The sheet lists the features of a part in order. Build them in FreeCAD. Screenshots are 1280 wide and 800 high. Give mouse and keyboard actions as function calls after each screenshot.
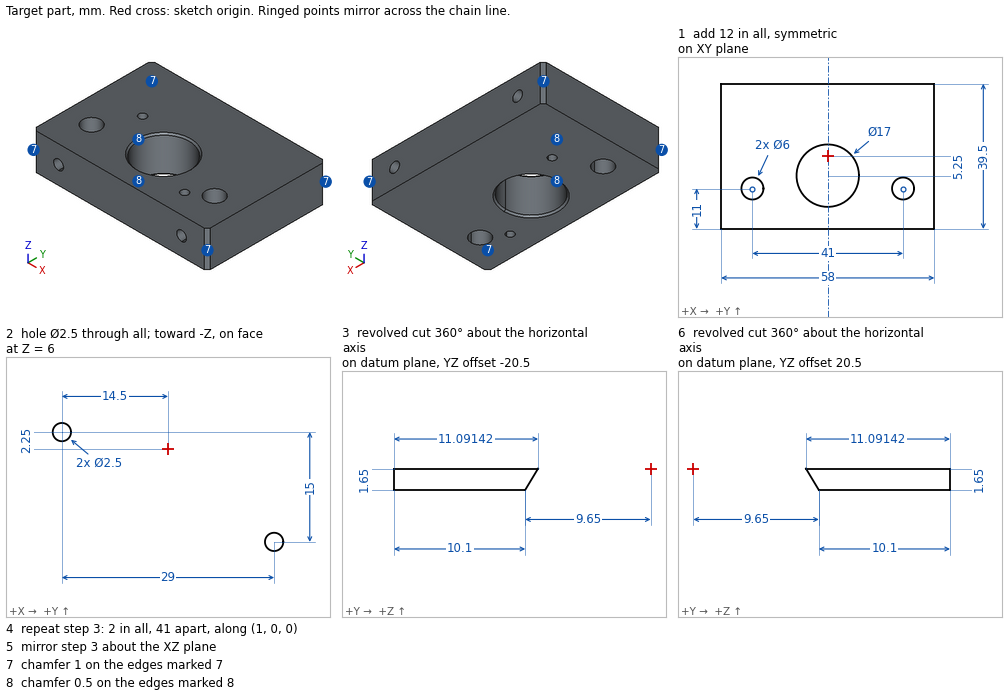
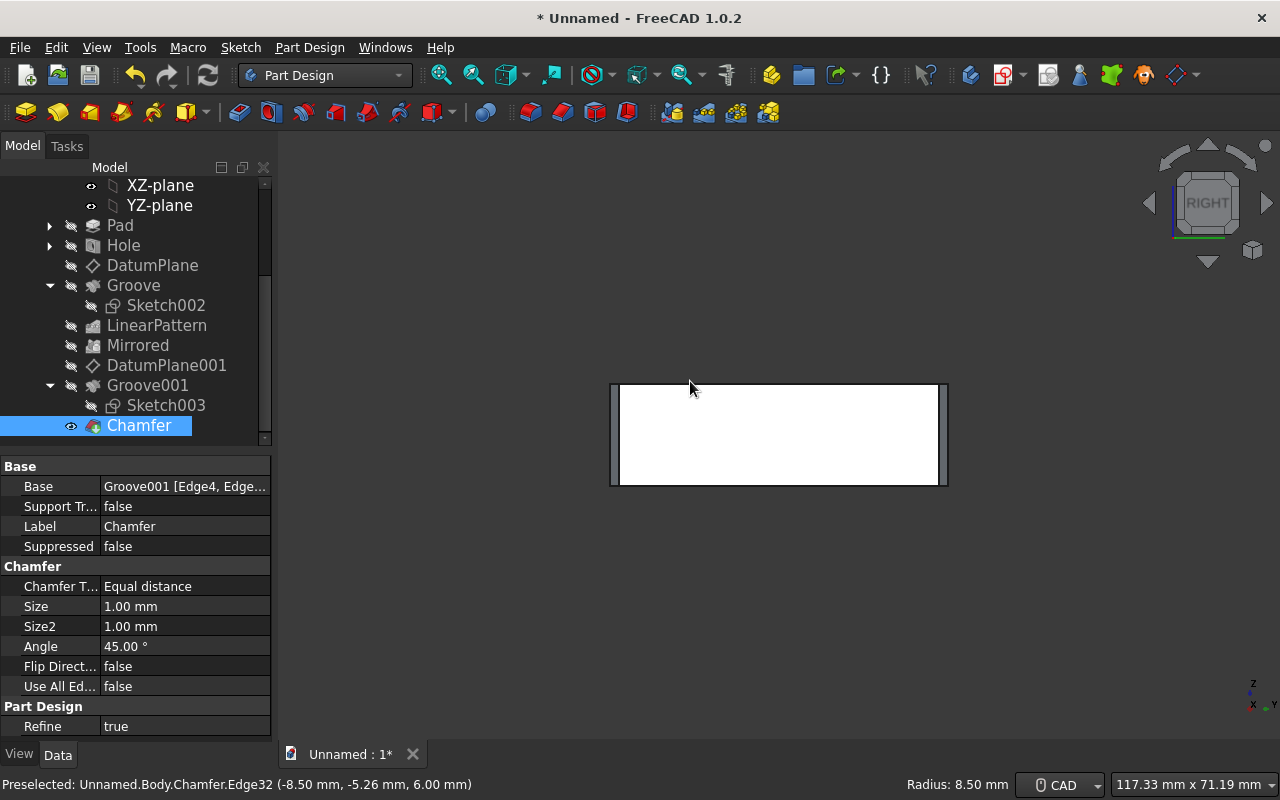
key(v)
key(f)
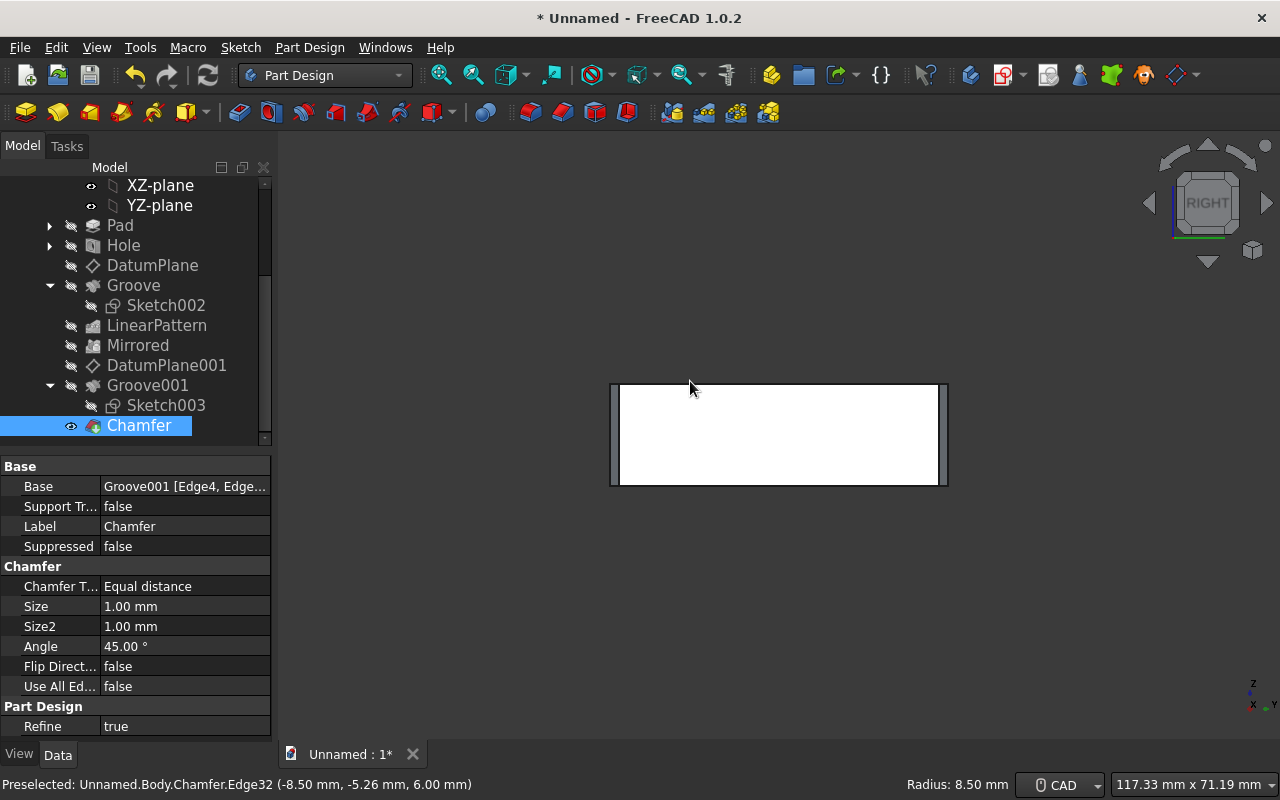
key(5)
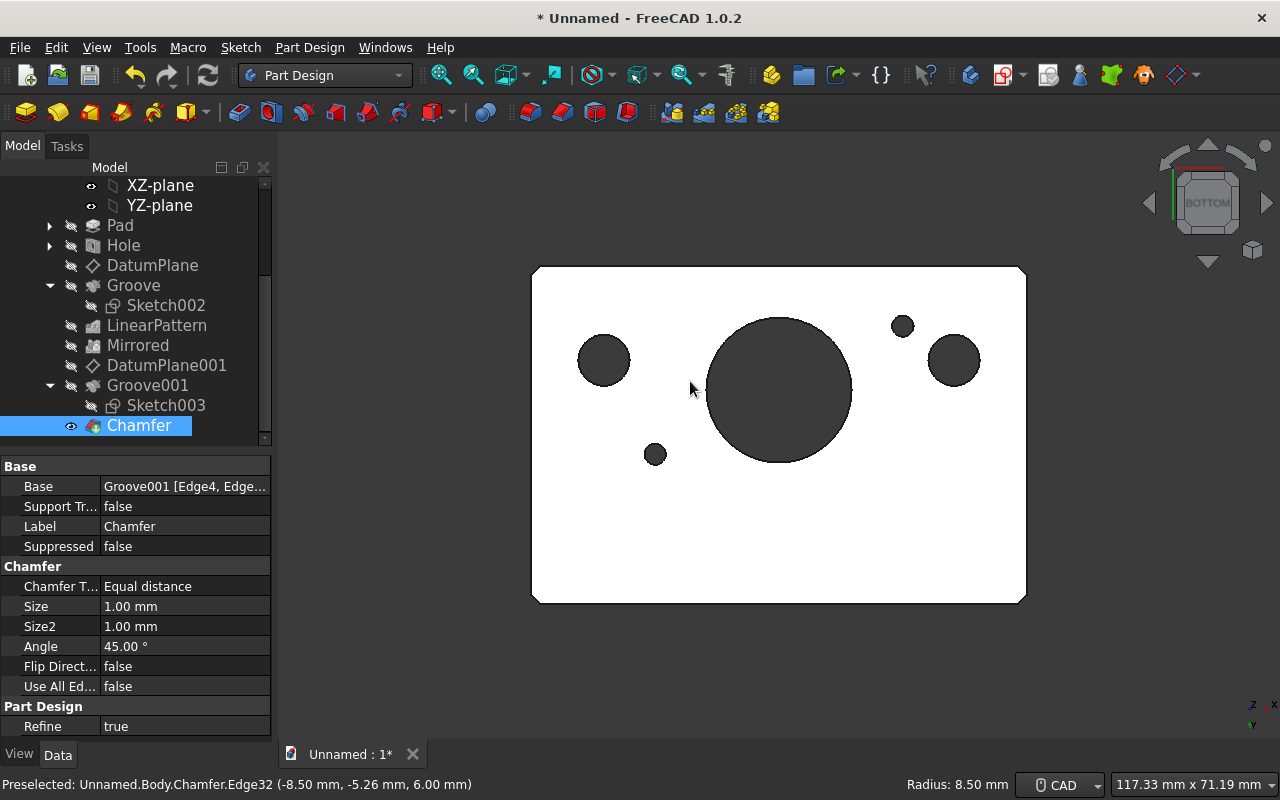
click(706, 389, ctrl)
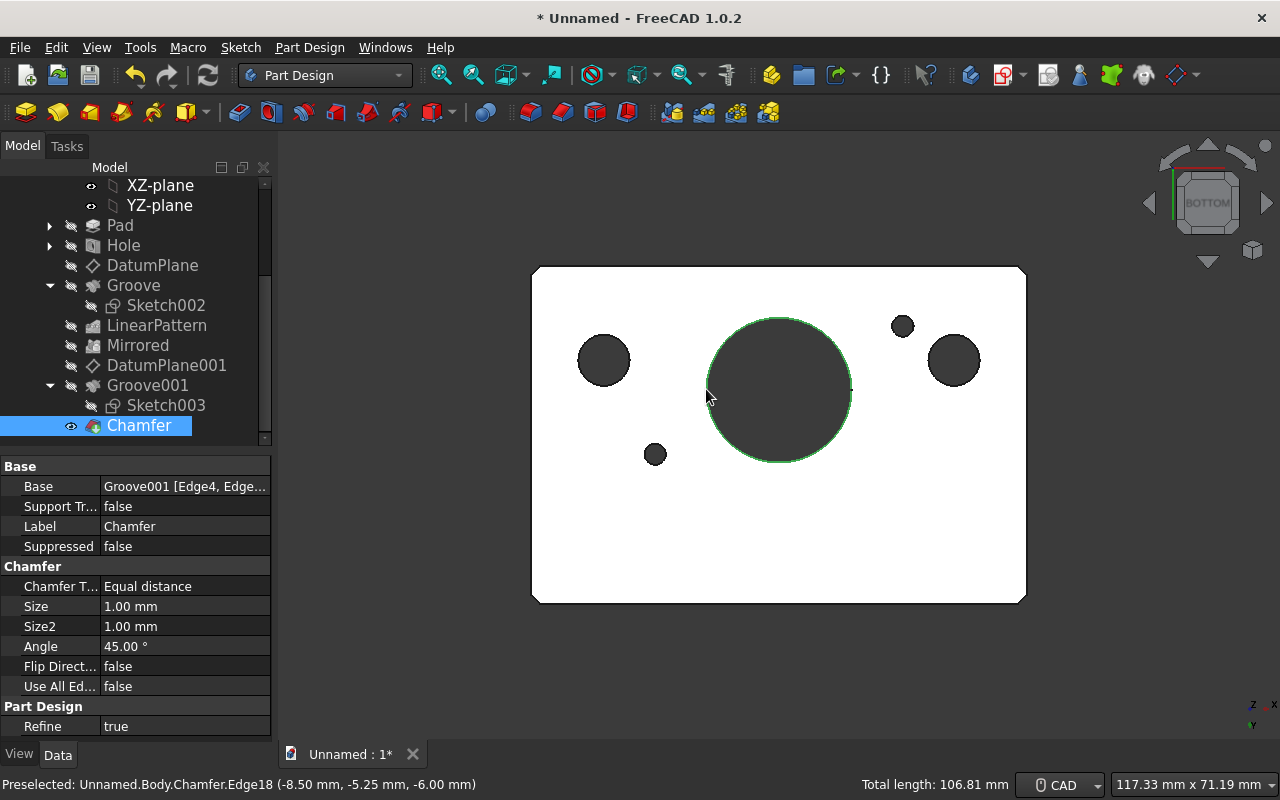
click(564, 112)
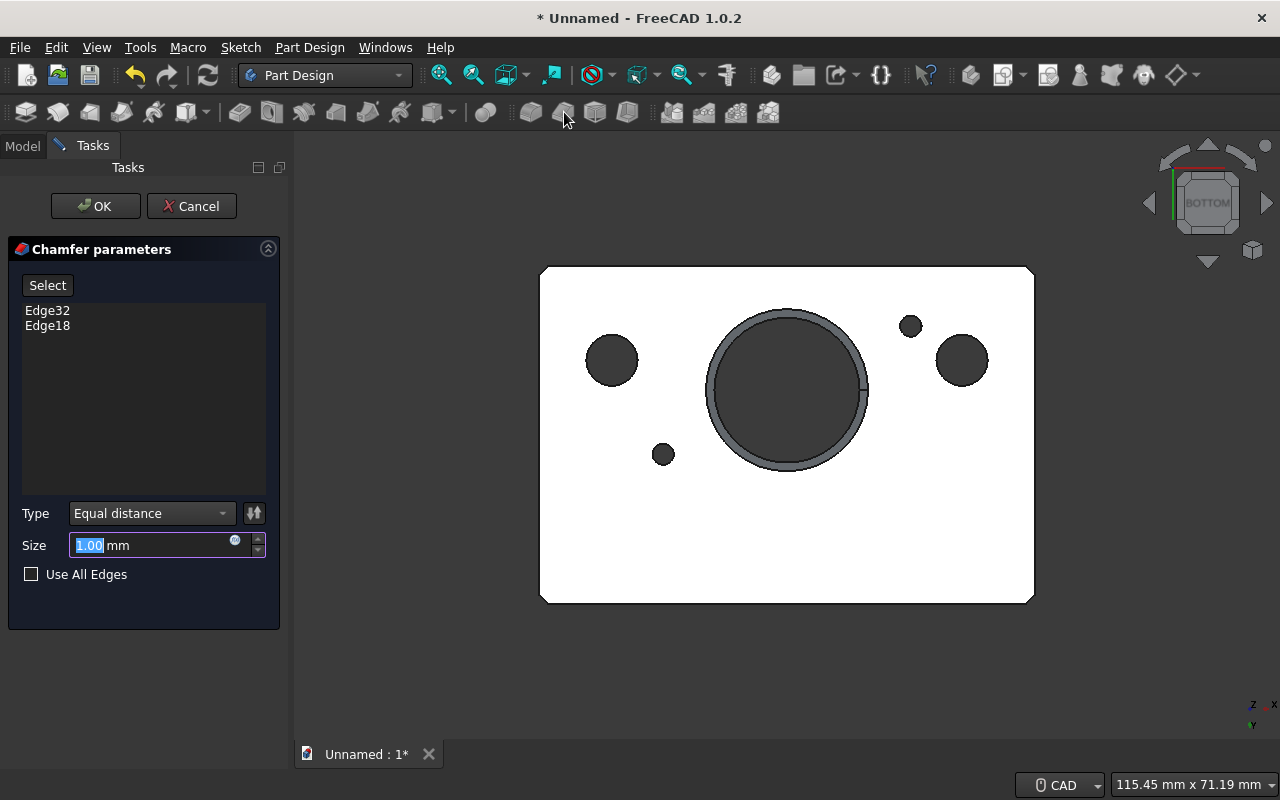
text(0.5)
key(Tab)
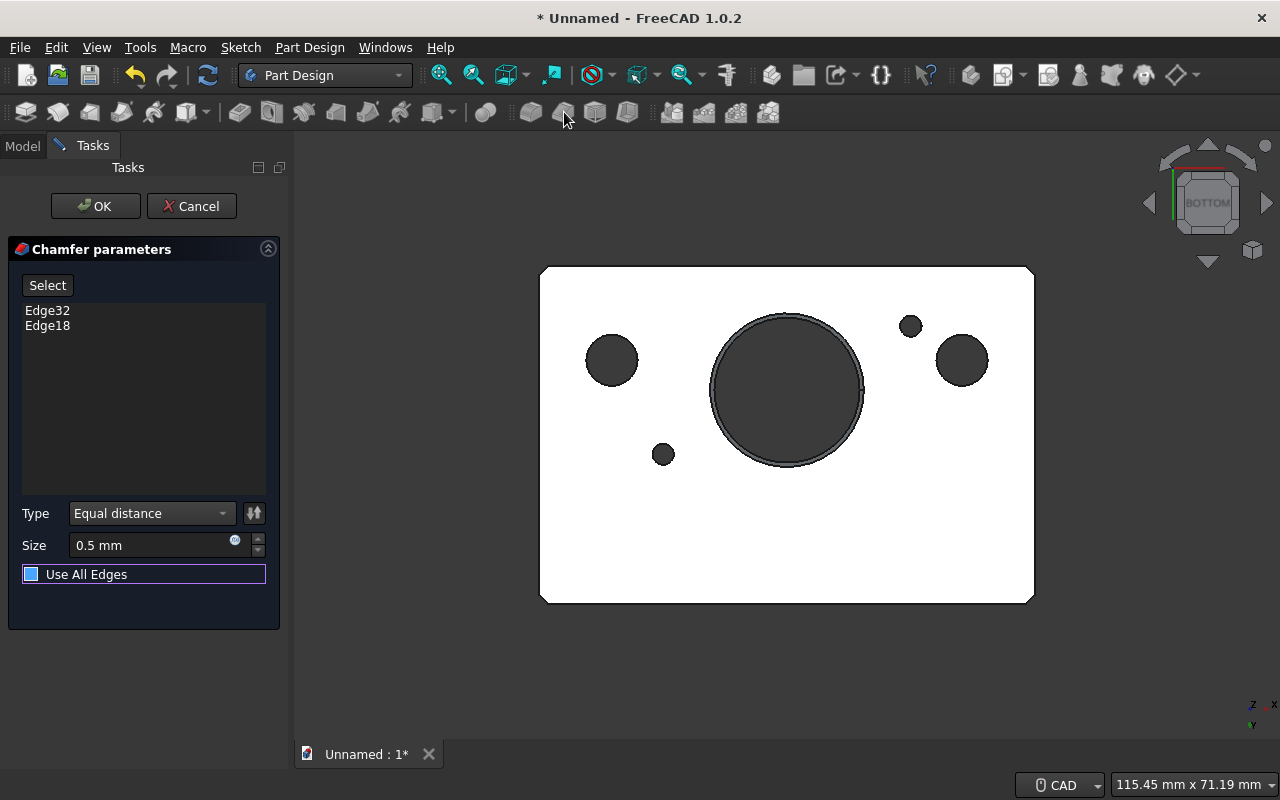
click(96, 206)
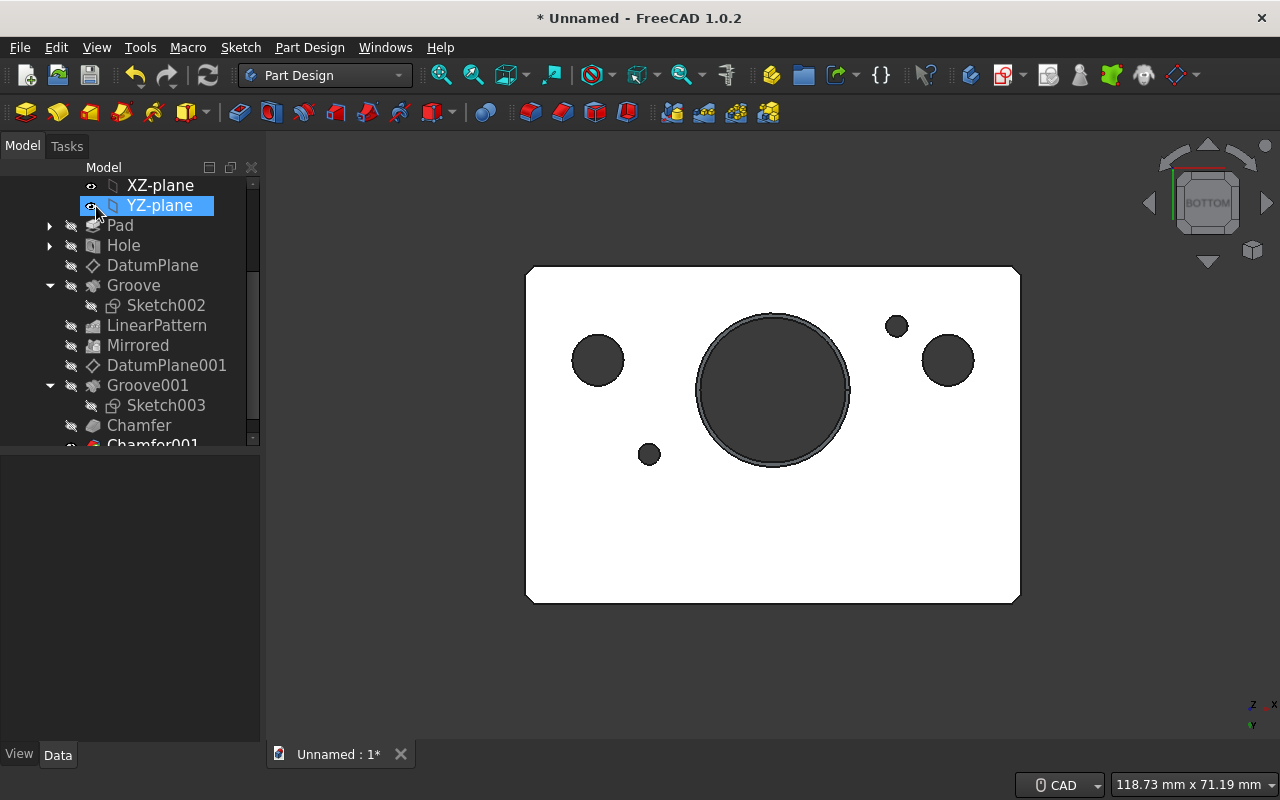
key(0)